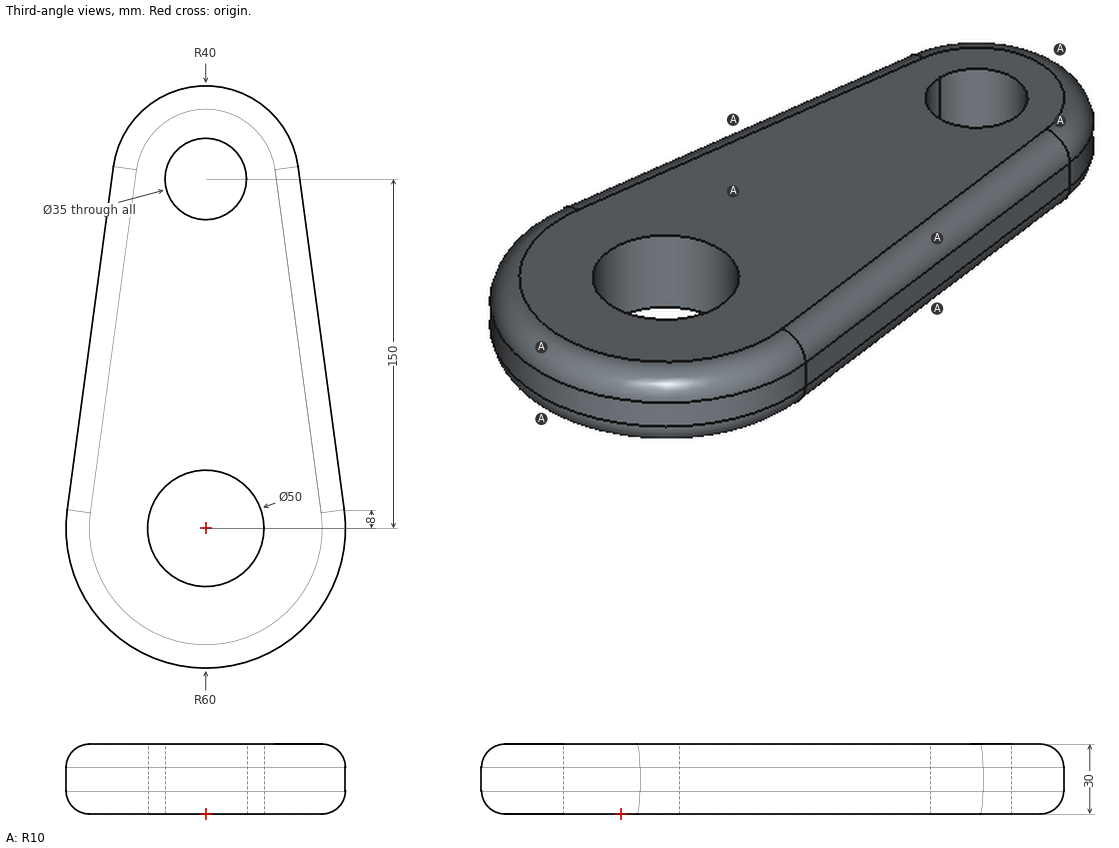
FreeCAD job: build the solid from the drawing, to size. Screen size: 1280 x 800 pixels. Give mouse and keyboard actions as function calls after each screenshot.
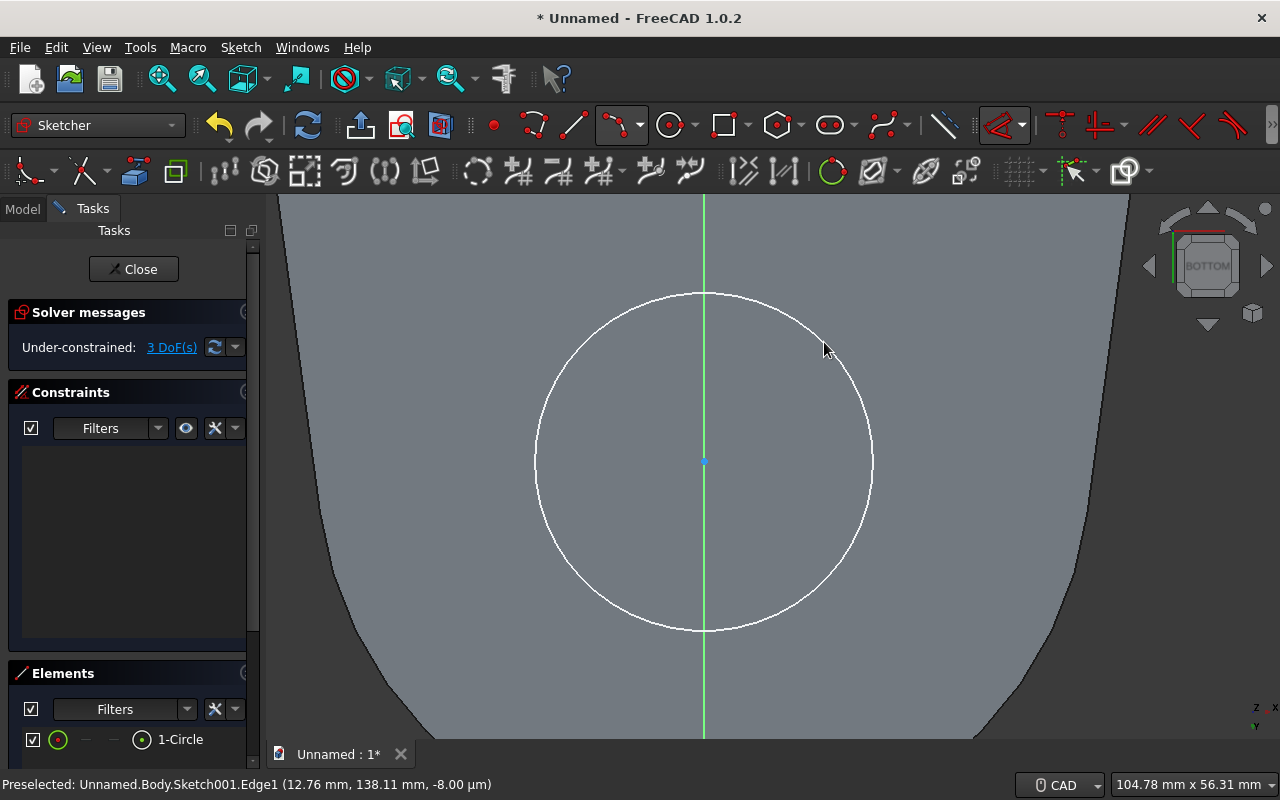
click(704, 462)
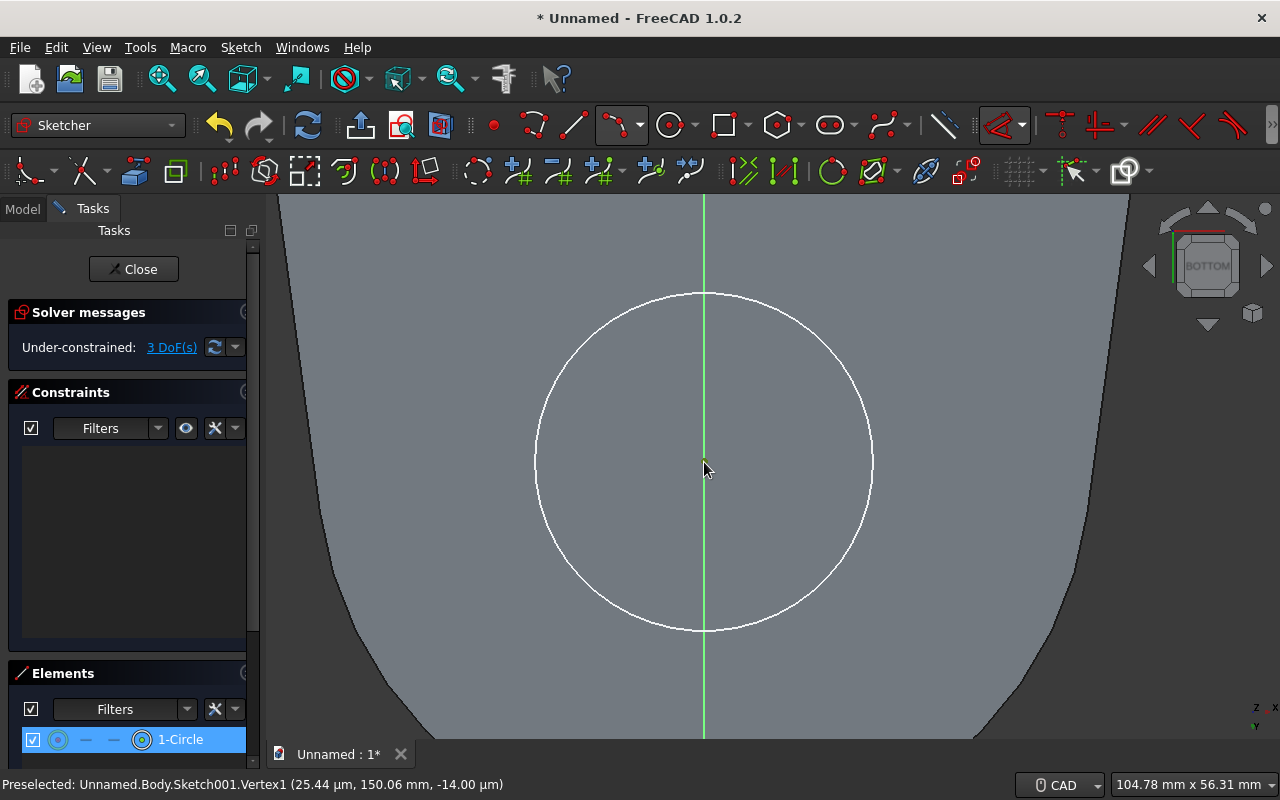
click(704, 676)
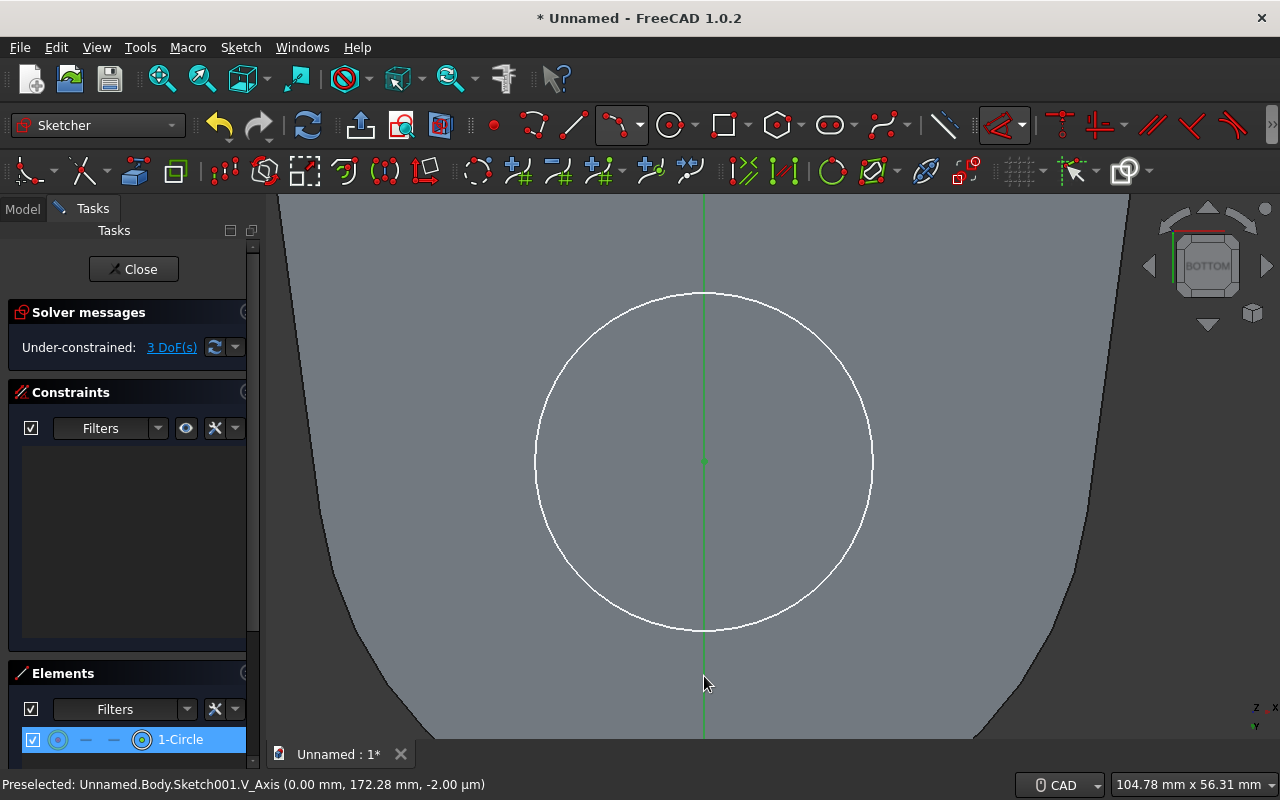
click(1060, 126)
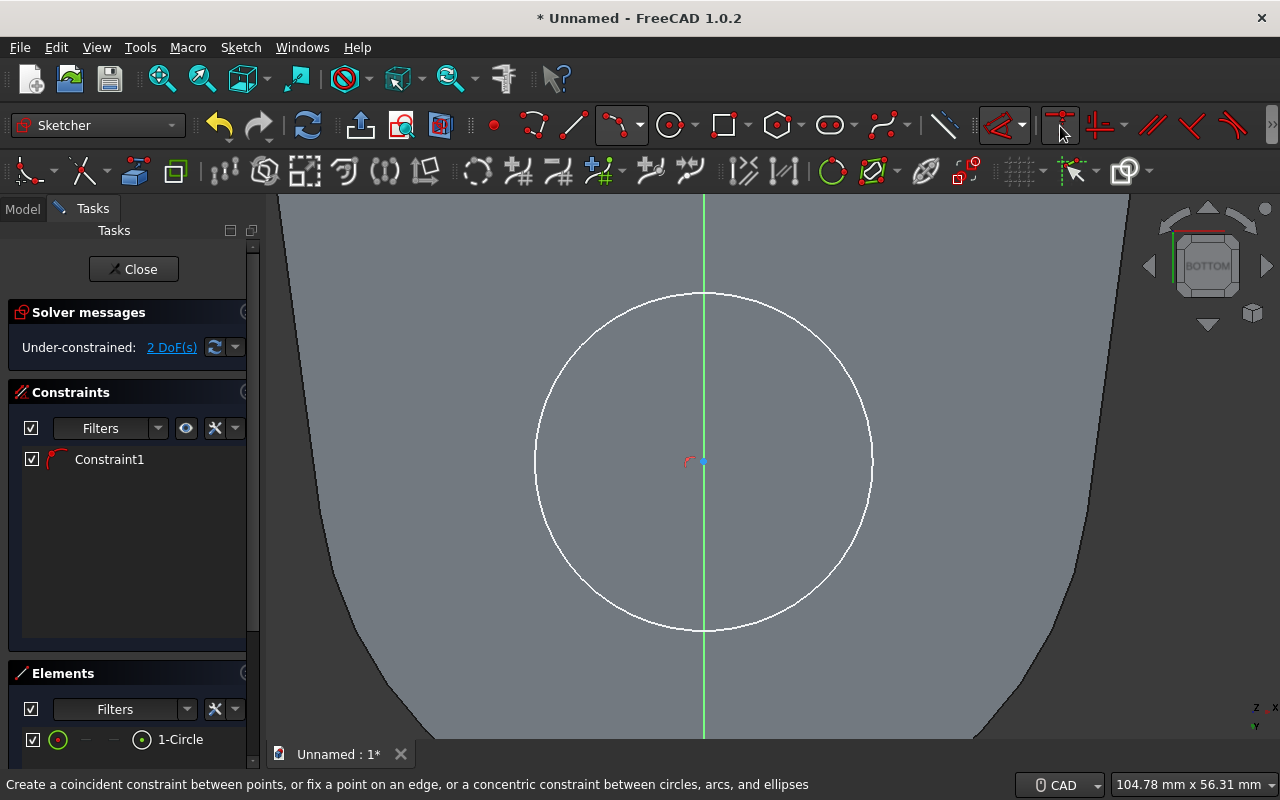
click(823, 342)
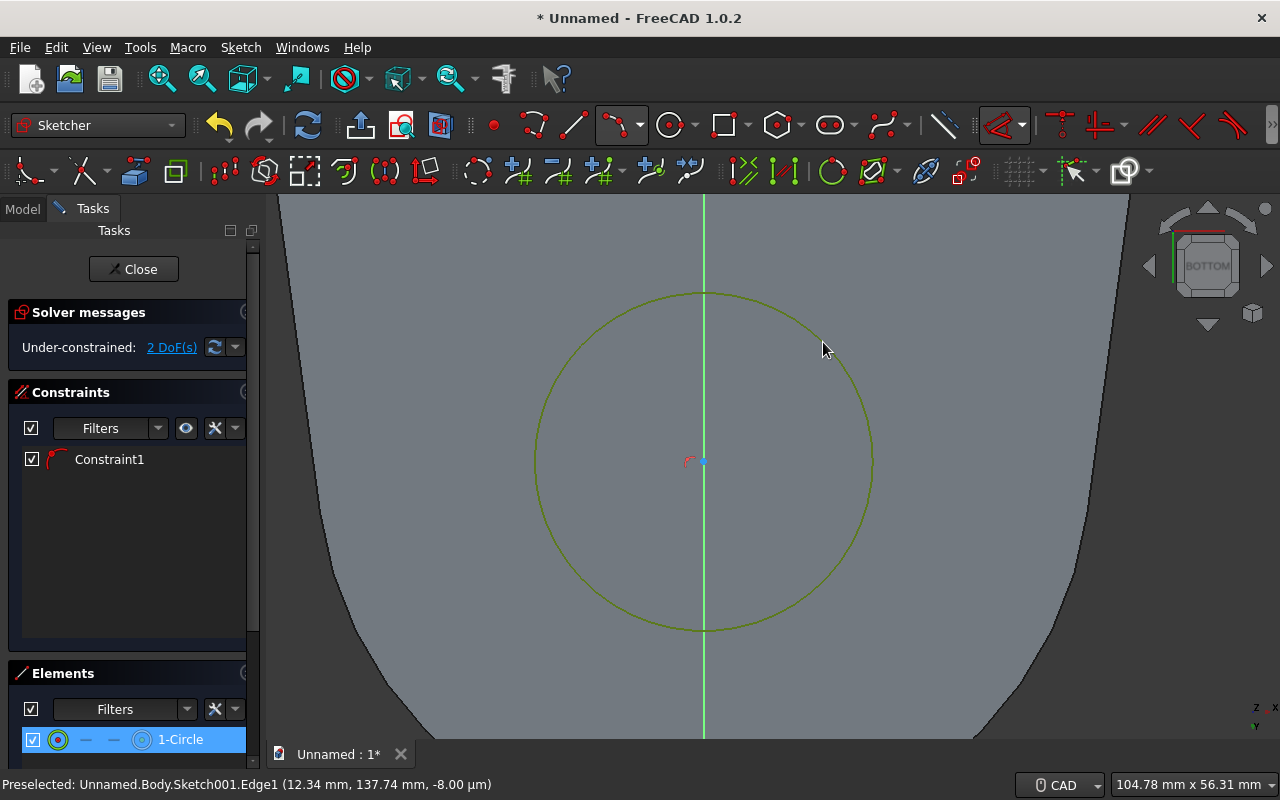
click(1024, 126)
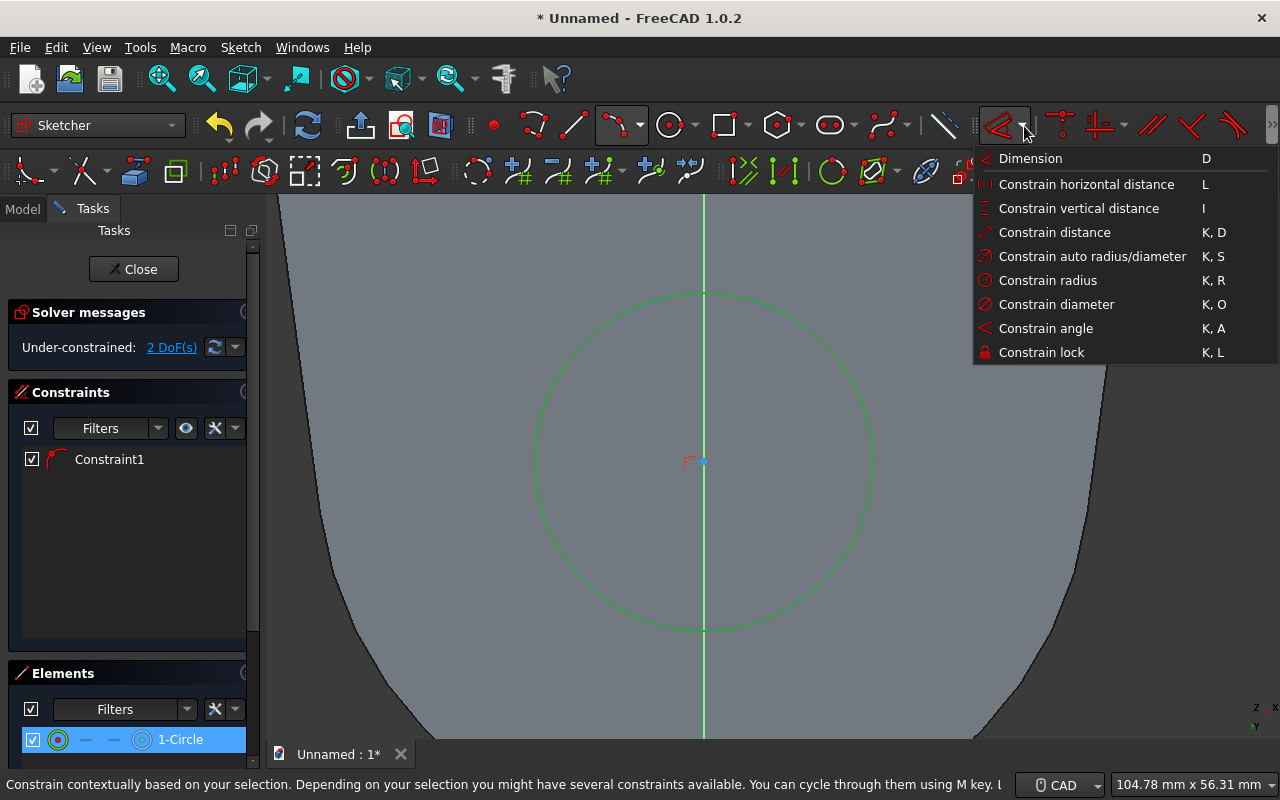
click(1126, 304)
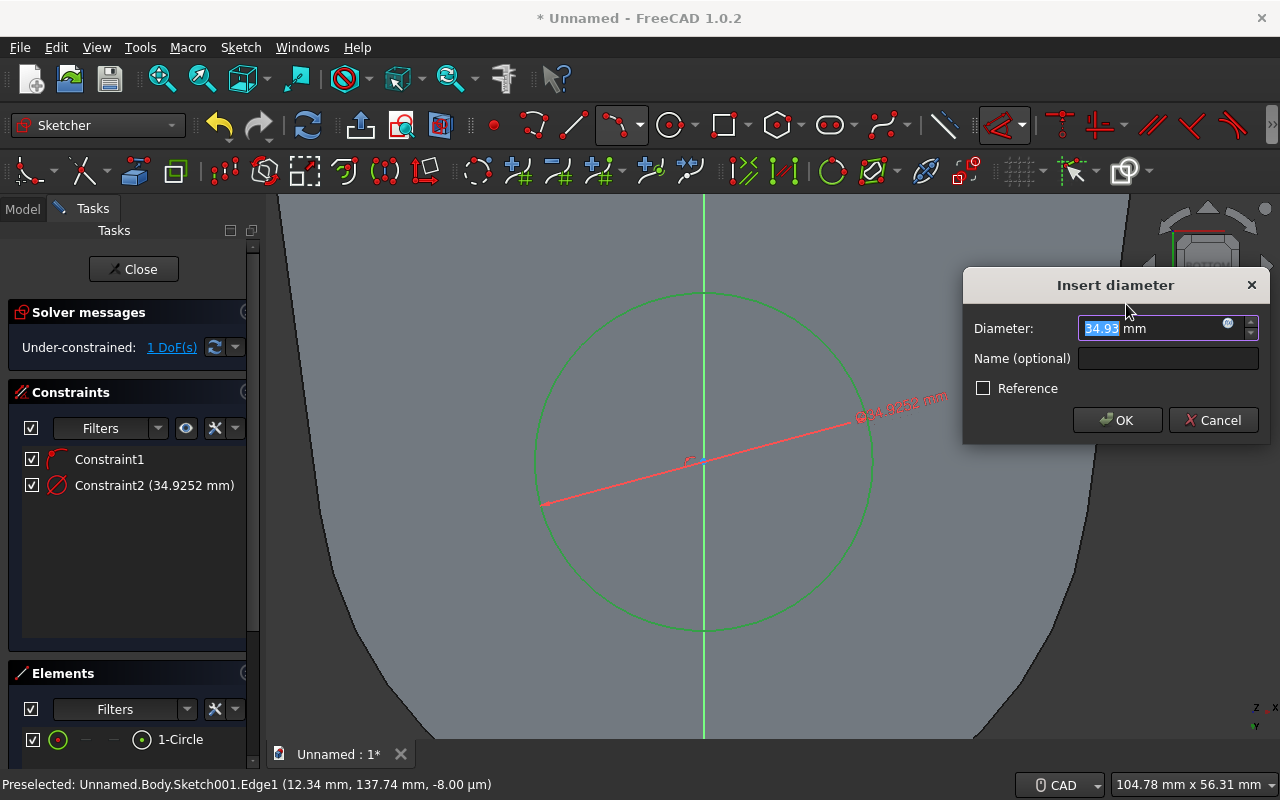
text(35)
key(Return)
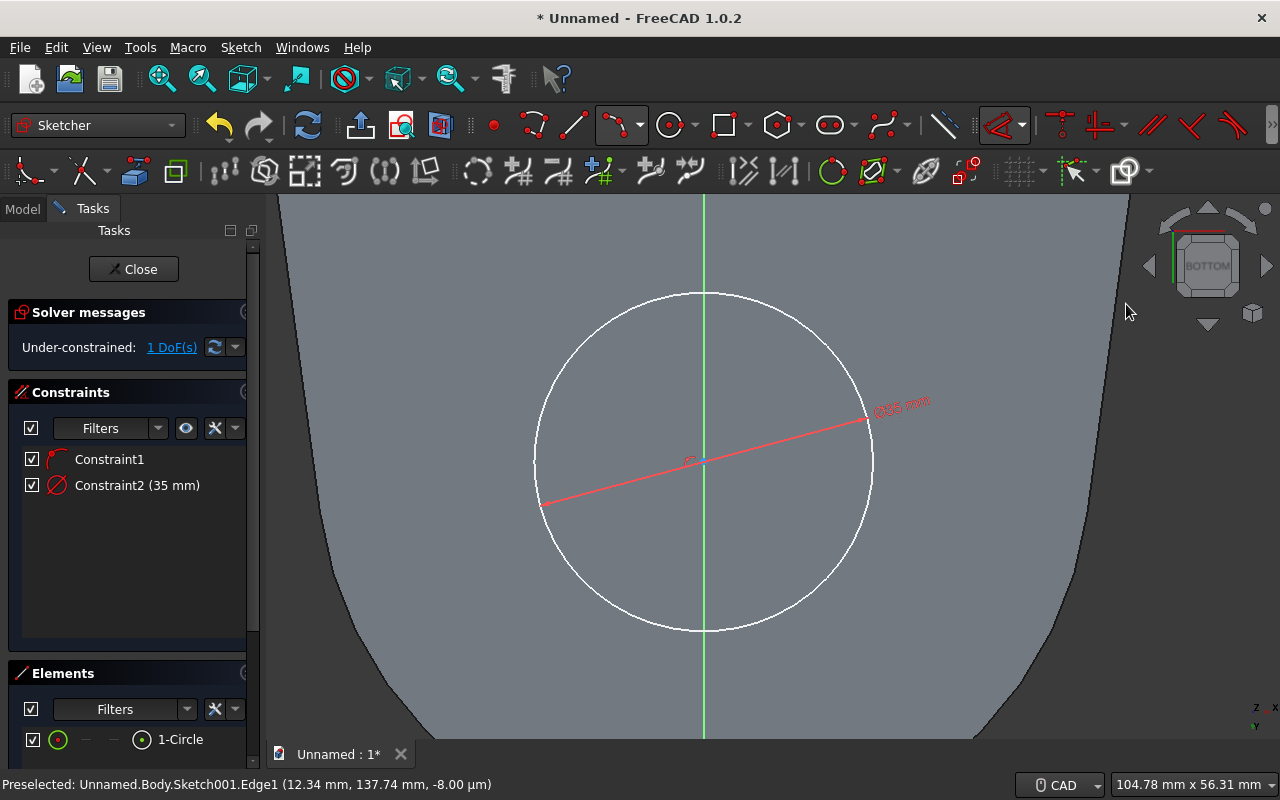
click(704, 462)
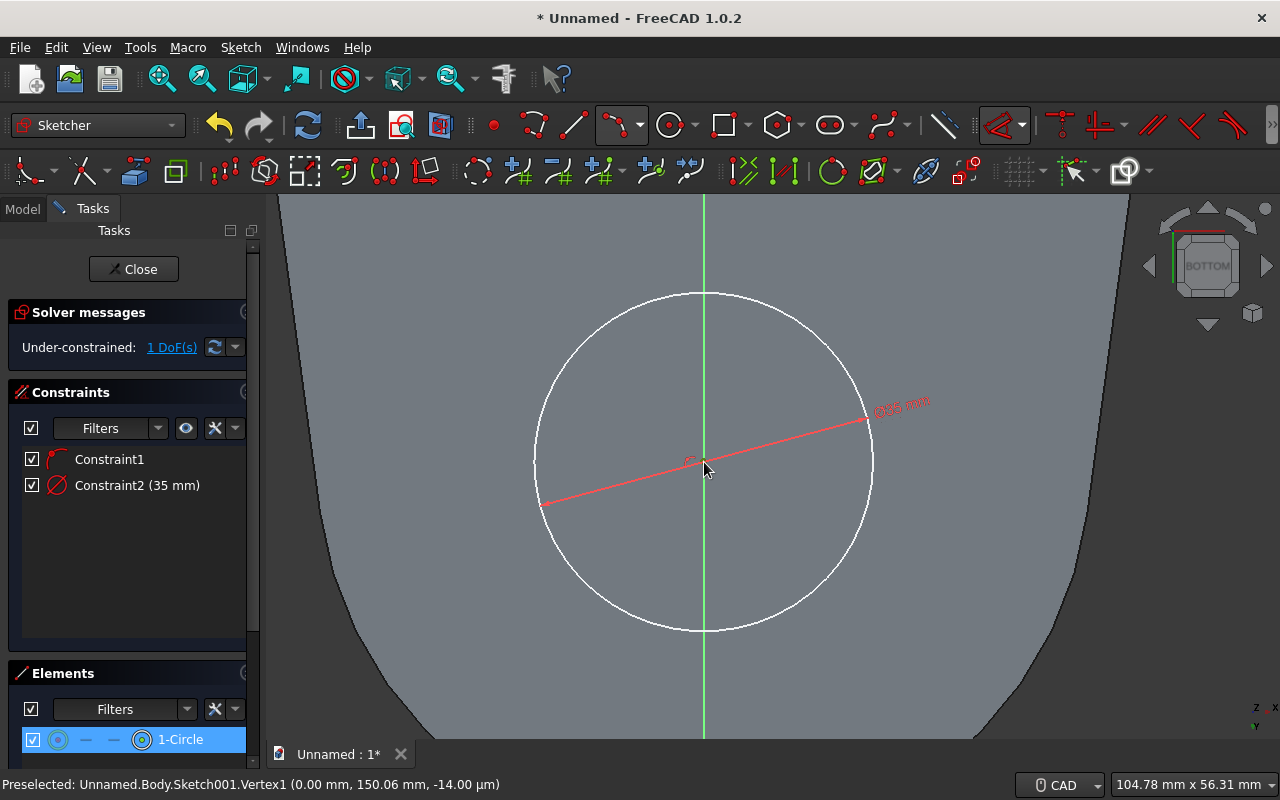
click(1024, 126)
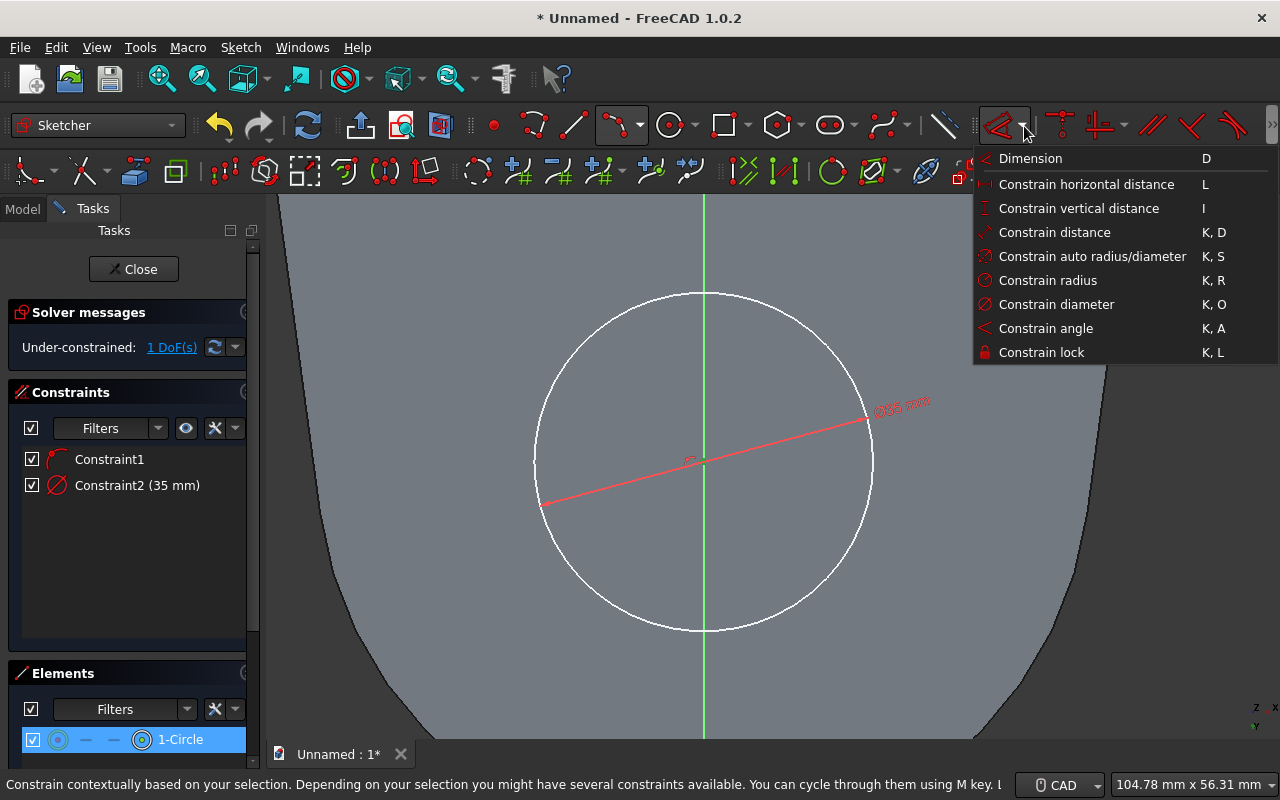
click(1126, 208)